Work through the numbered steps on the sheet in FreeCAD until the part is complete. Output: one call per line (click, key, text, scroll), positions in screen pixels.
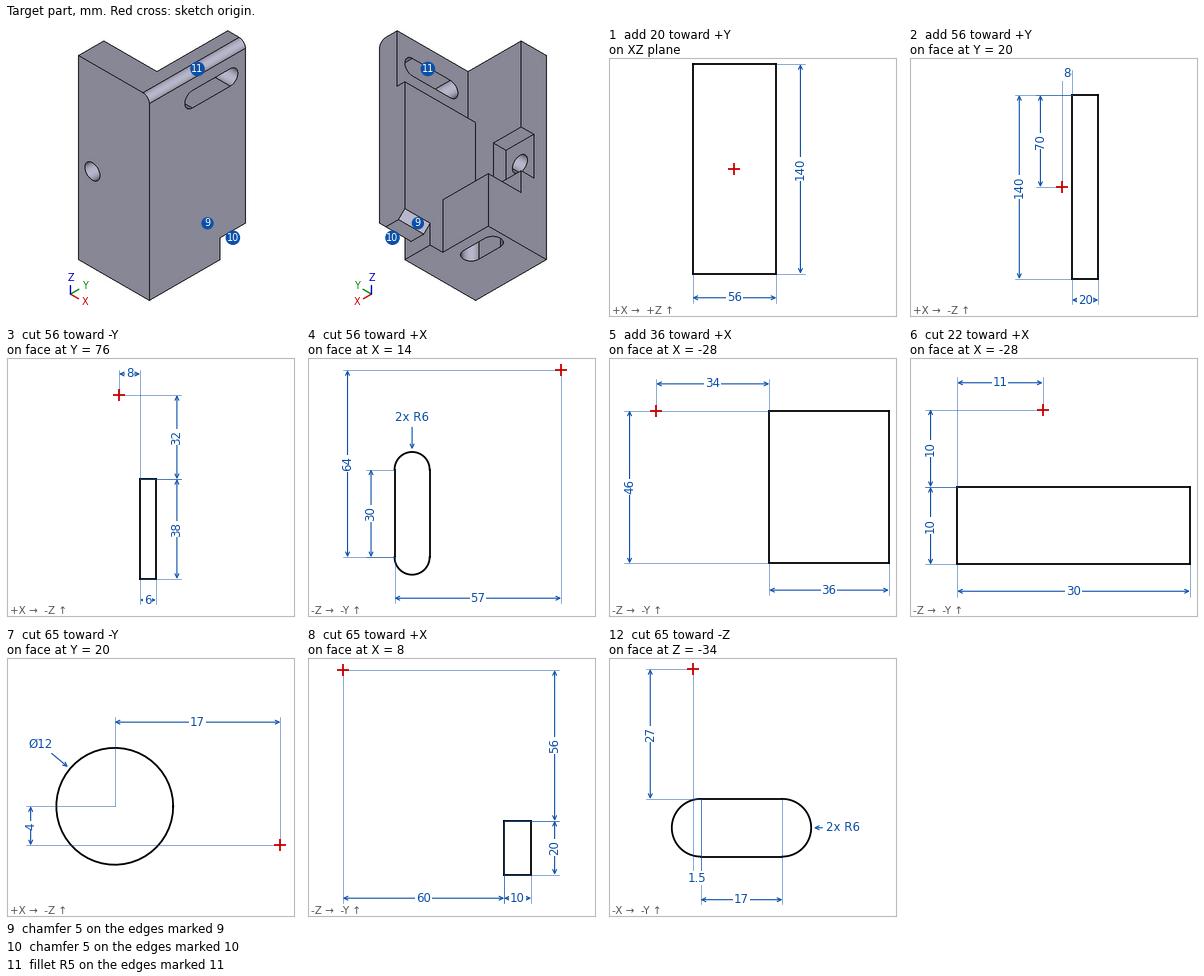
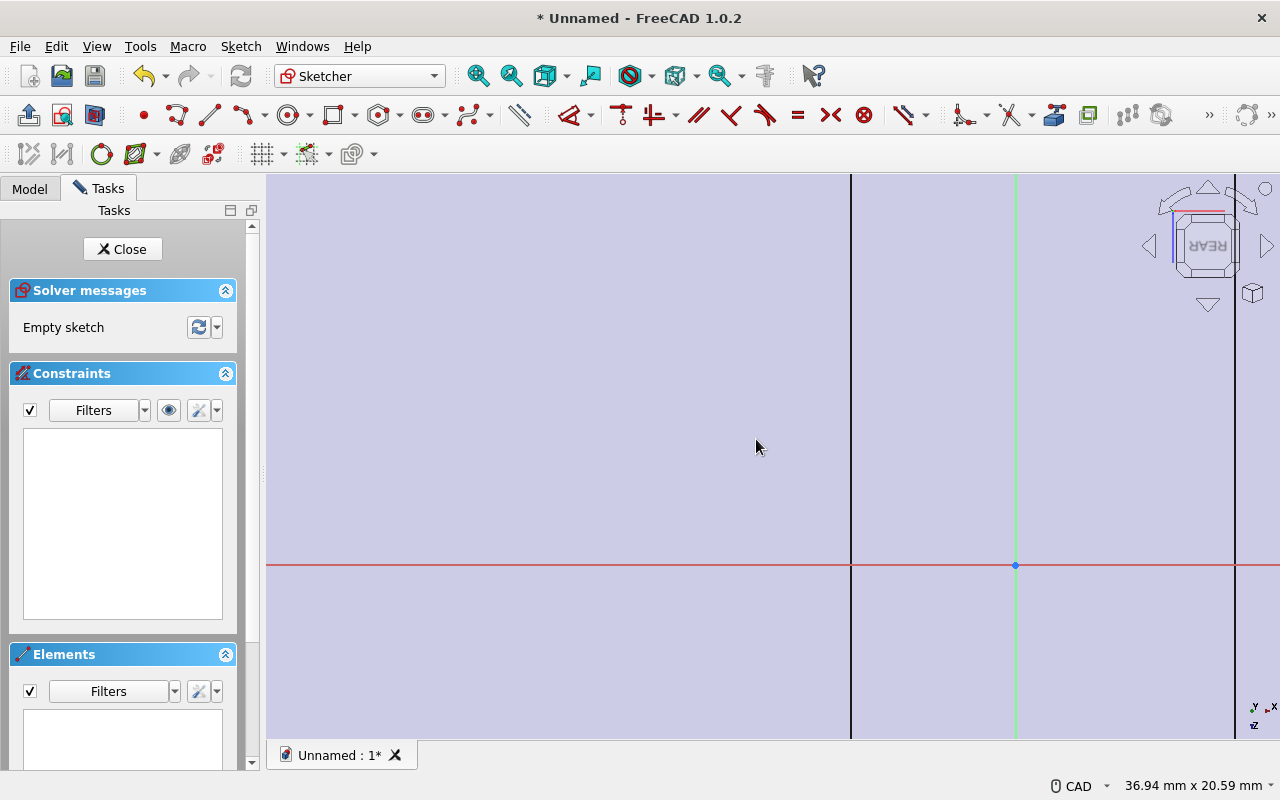
key(g)
key(c)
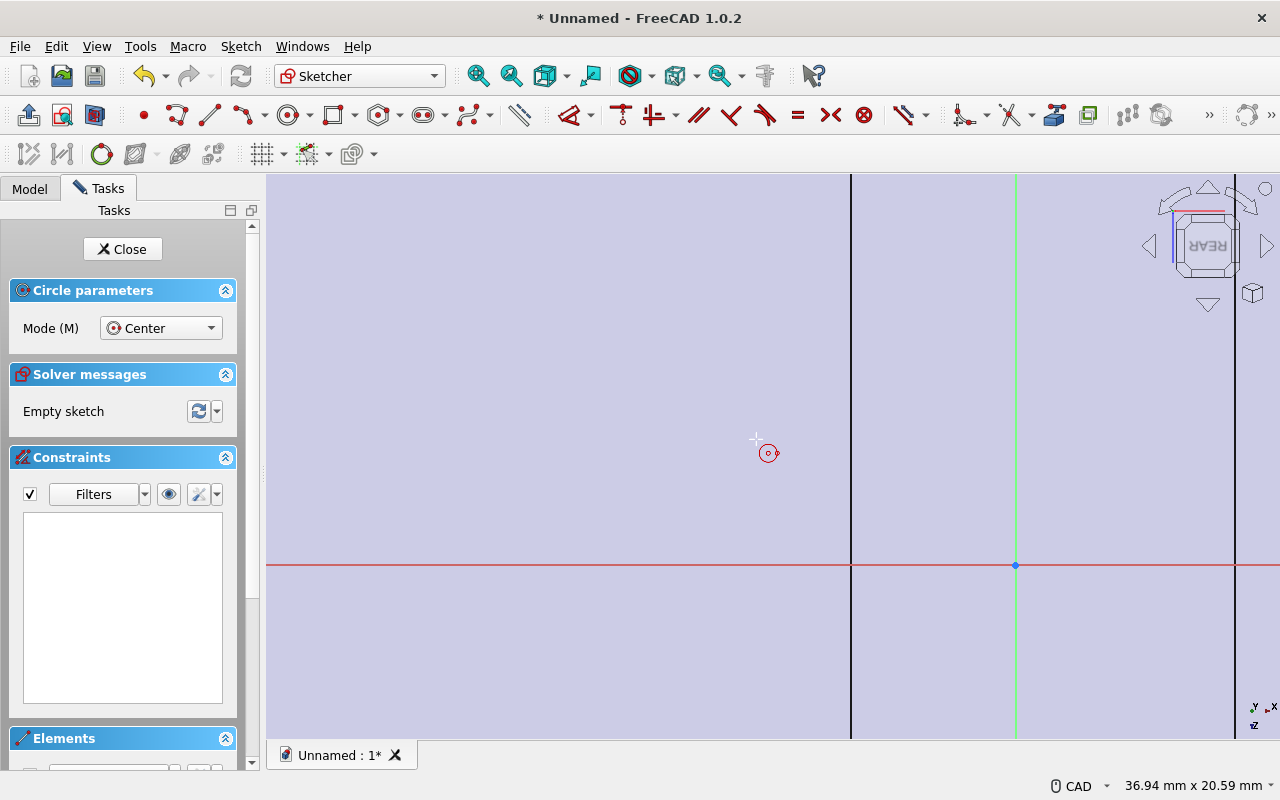
click(549, 456)
click(666, 339)
key(Escape)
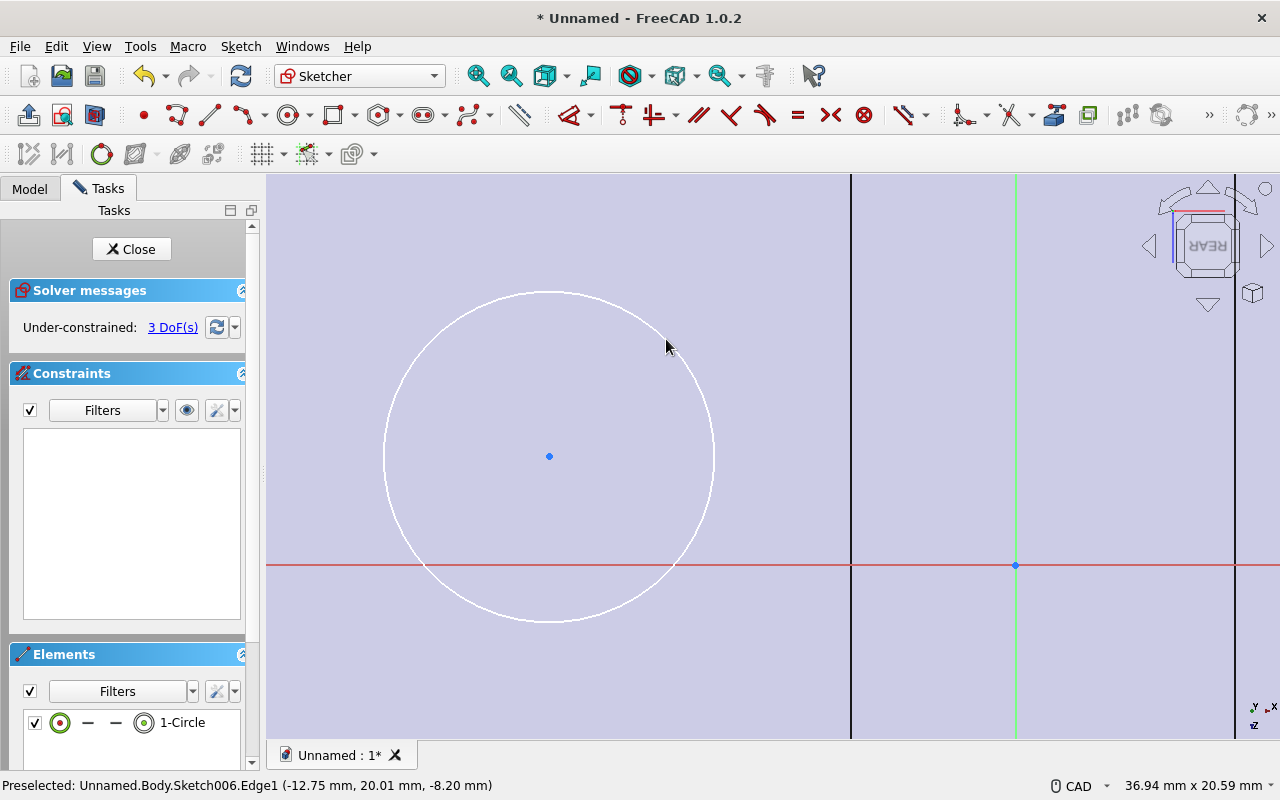
click(568, 116)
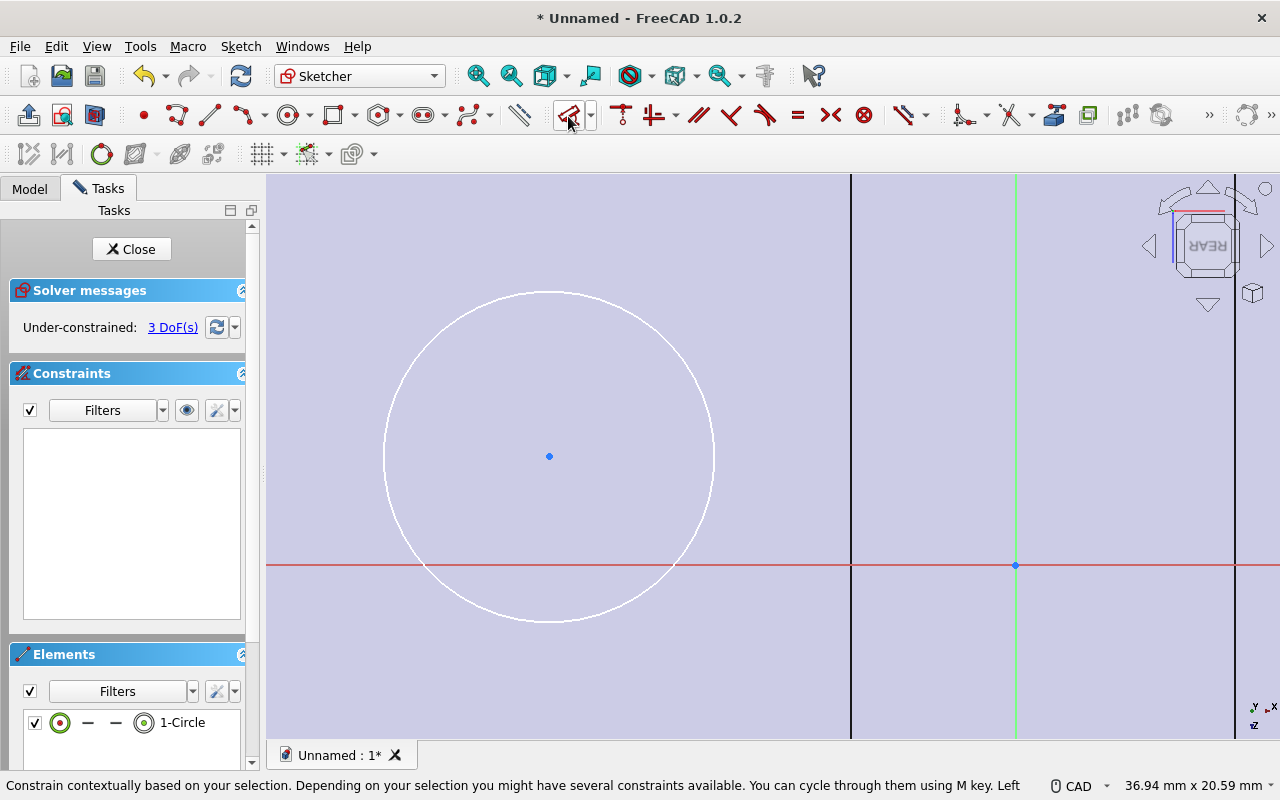
click(666, 340)
click(689, 317)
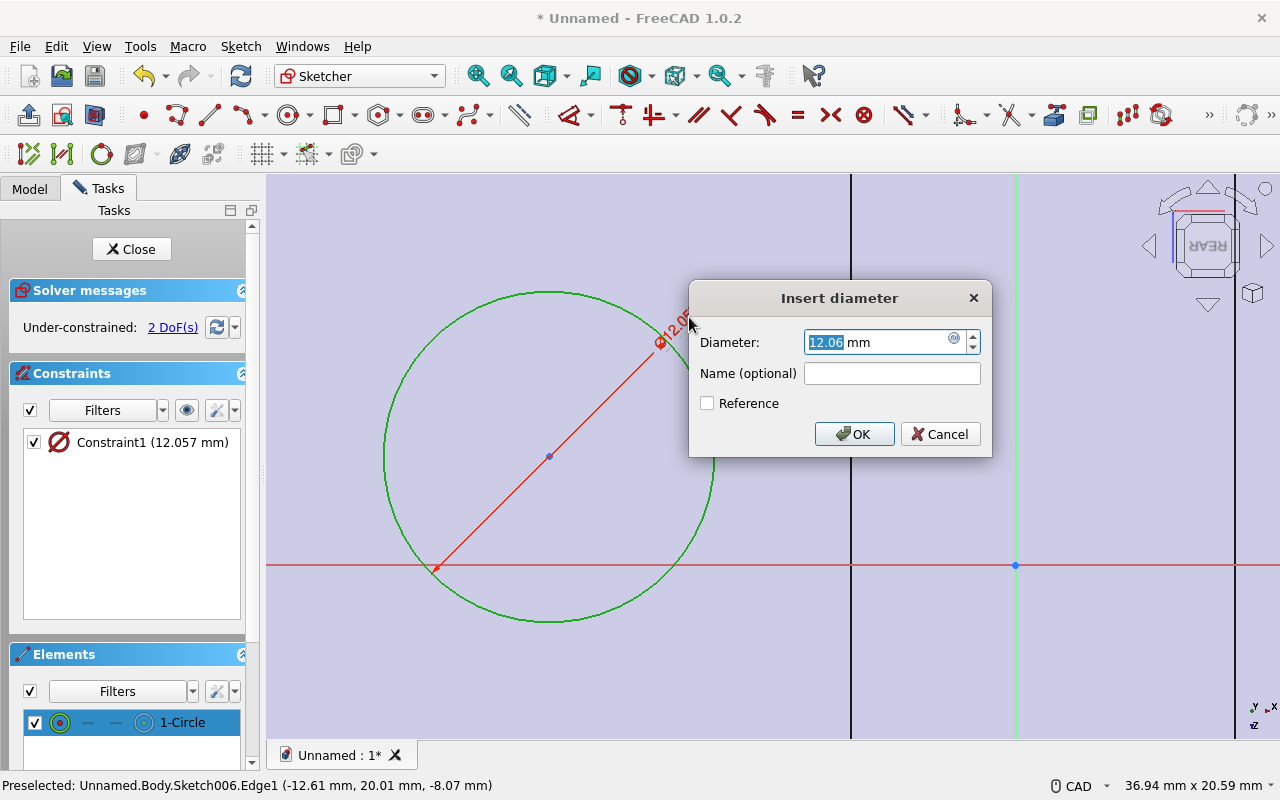
text(12)
key(Return)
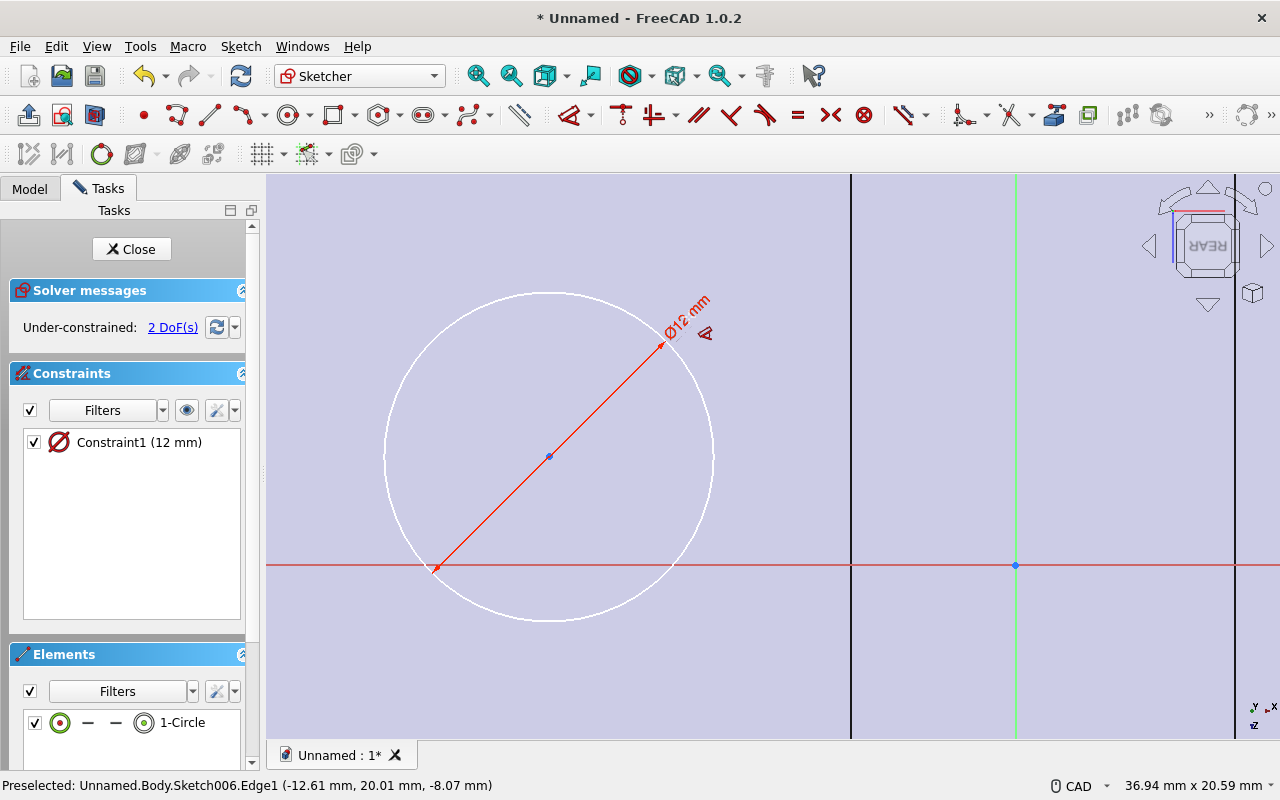
click(549, 457)
click(1050, 511)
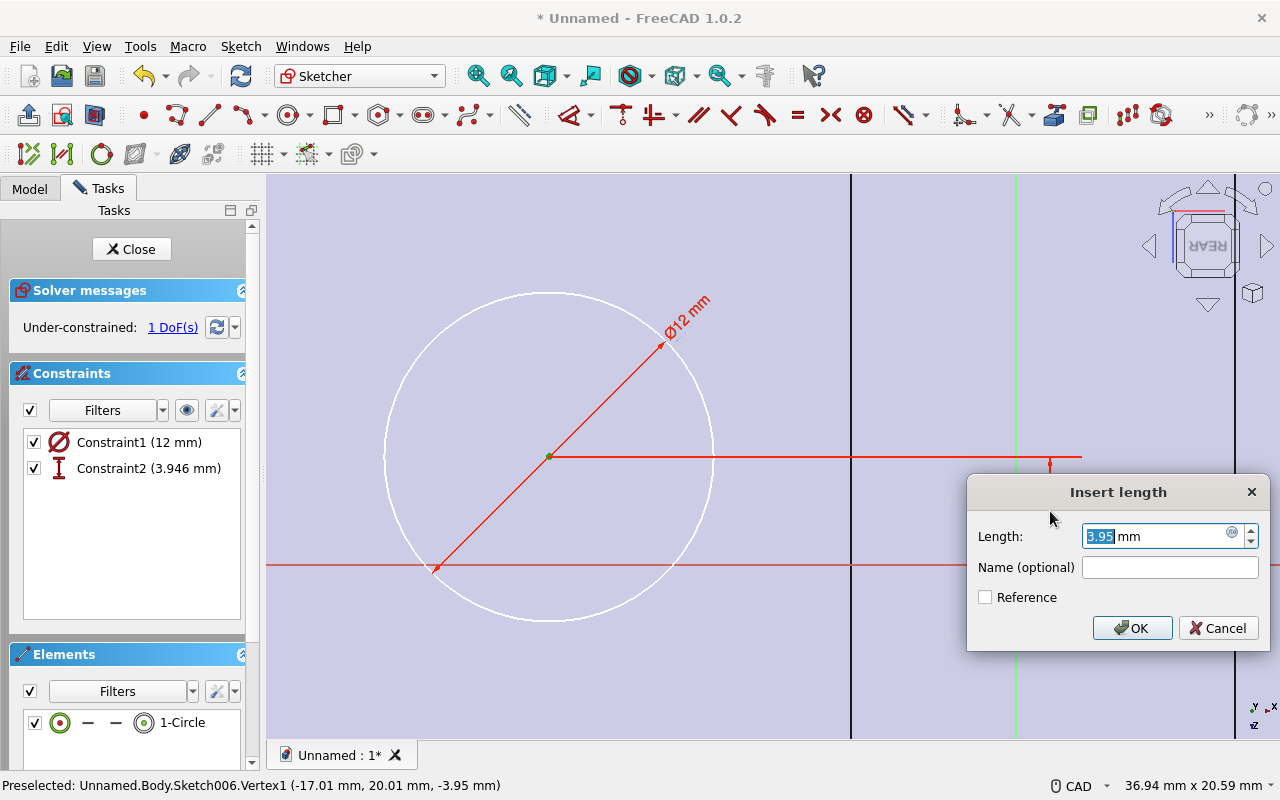
text(4)
key(Return)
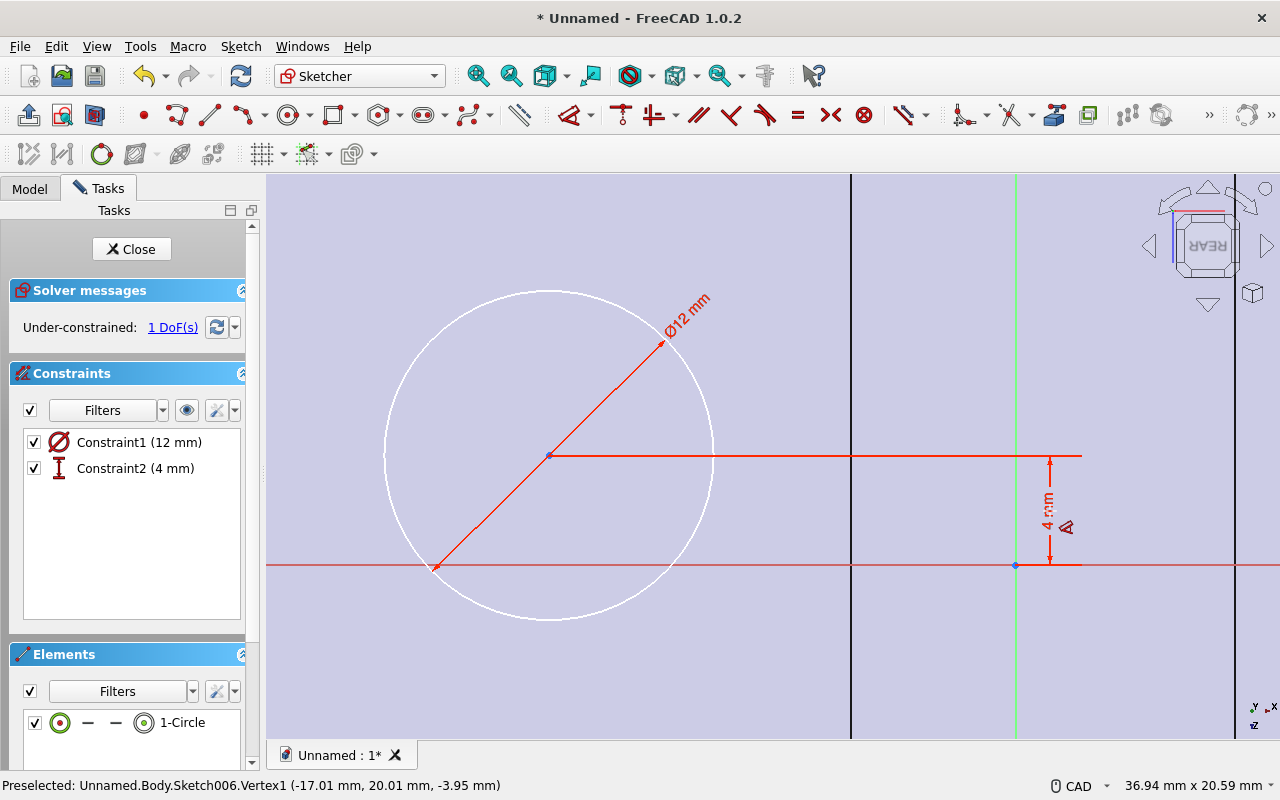
click(549, 456)
click(782, 599)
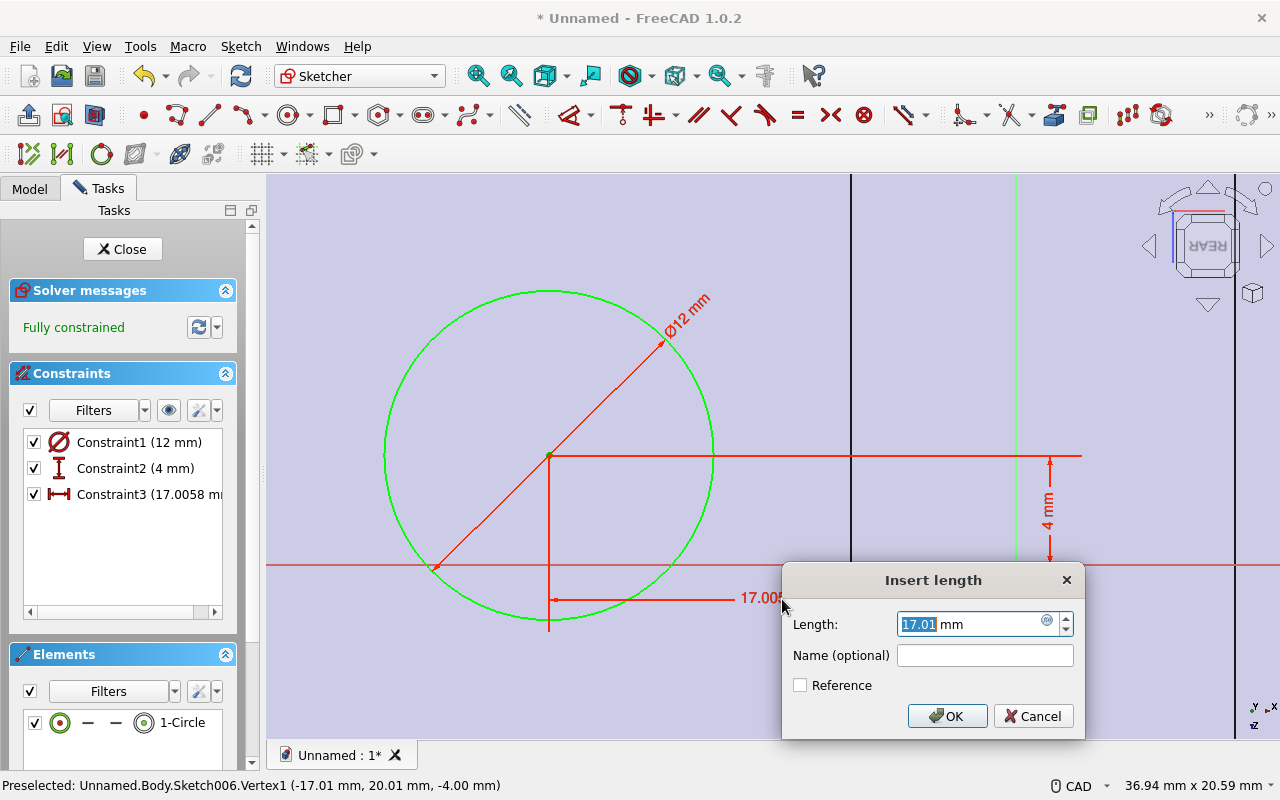
text(17)
key(Return)
key(Escape)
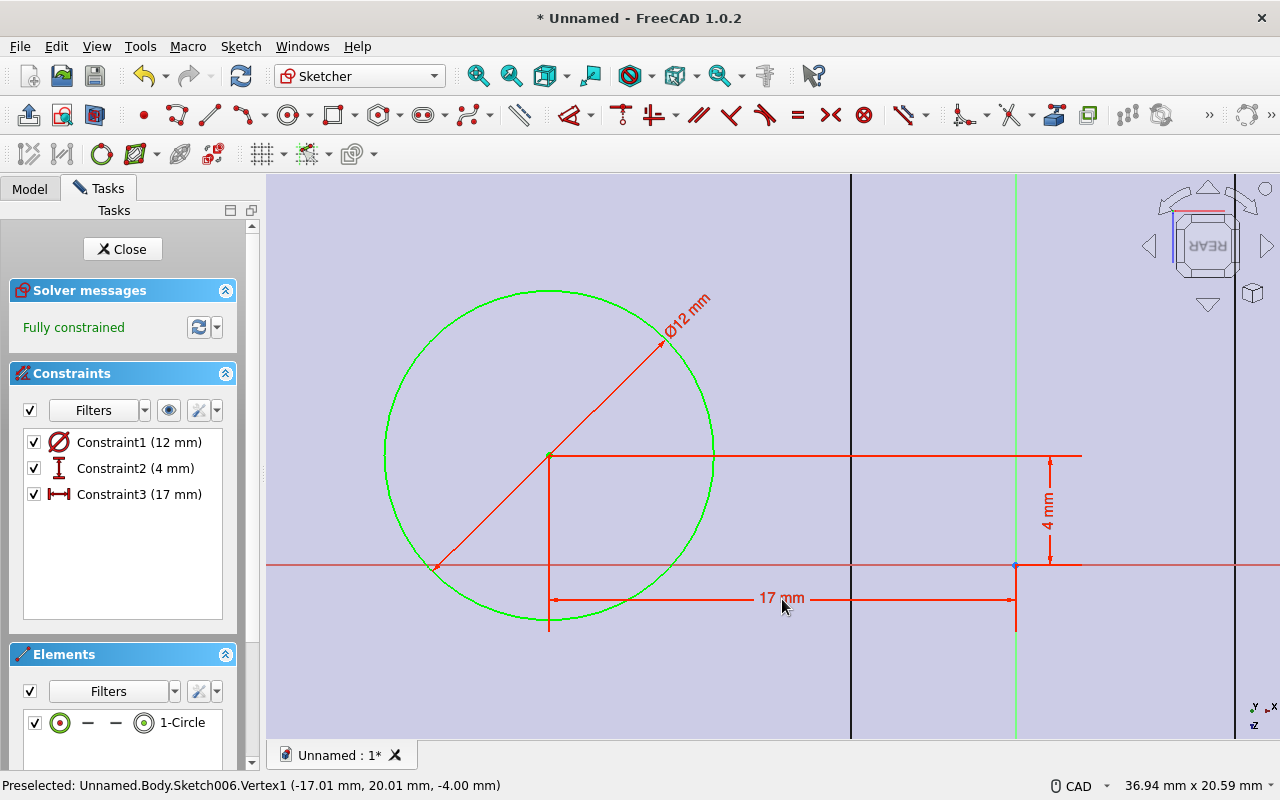
click(123, 249)